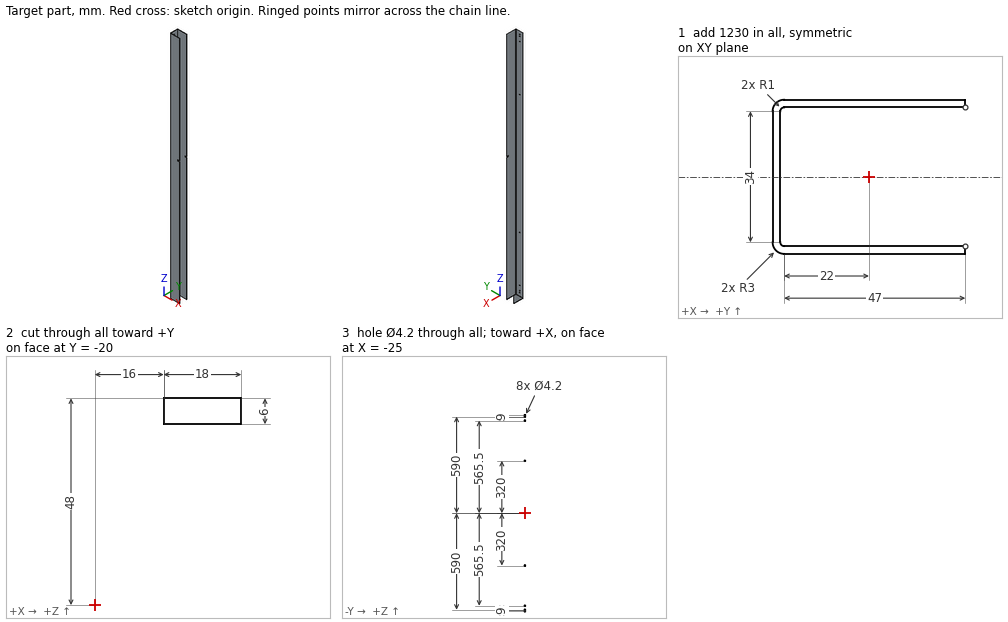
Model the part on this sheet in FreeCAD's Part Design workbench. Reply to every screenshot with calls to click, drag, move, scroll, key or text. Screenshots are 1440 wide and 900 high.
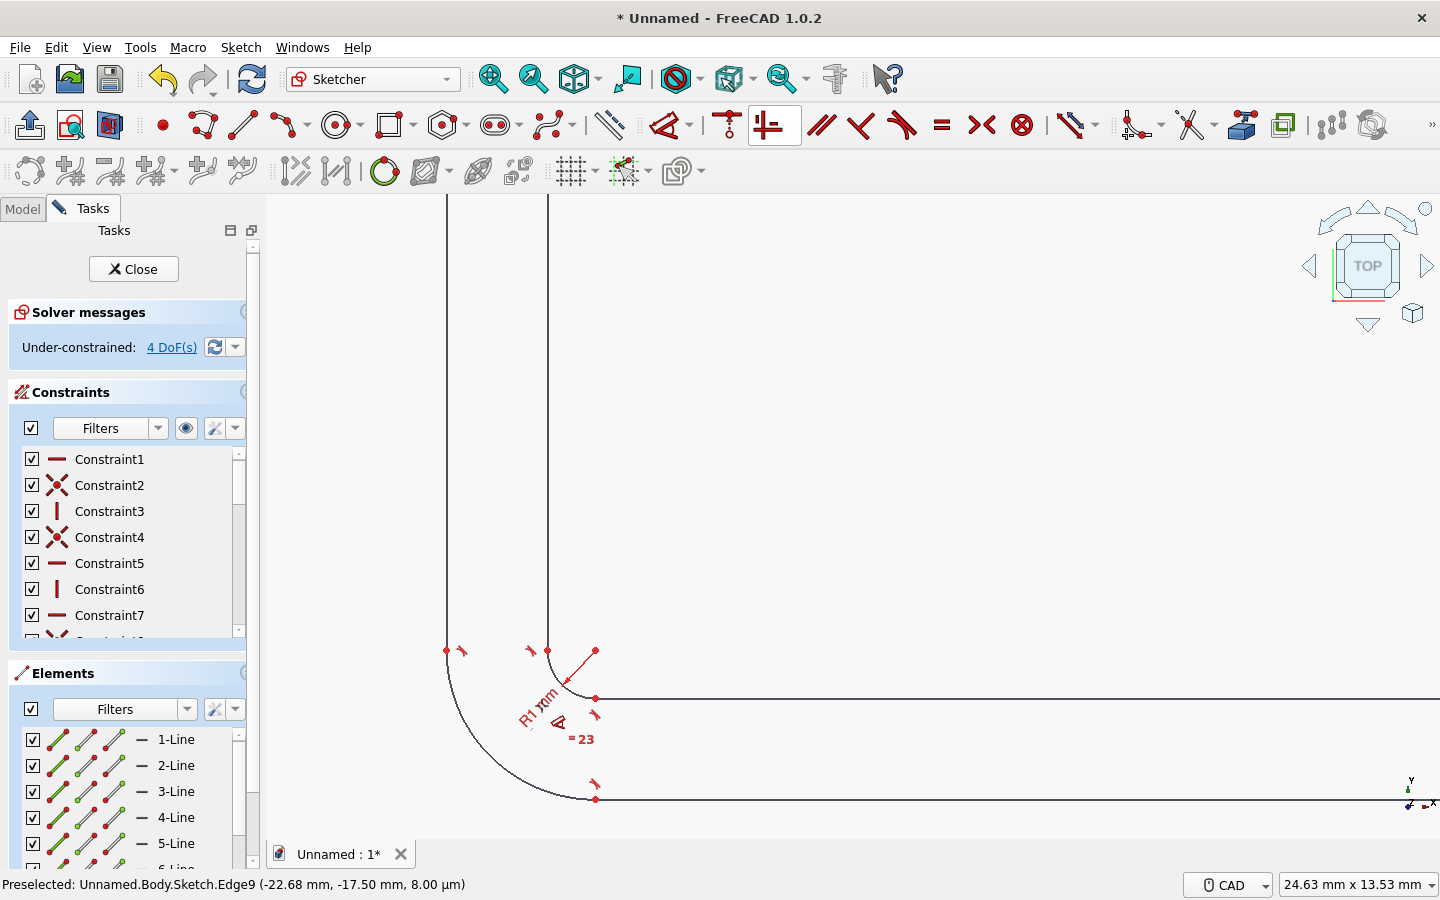
scroll(567, 686, down, 8)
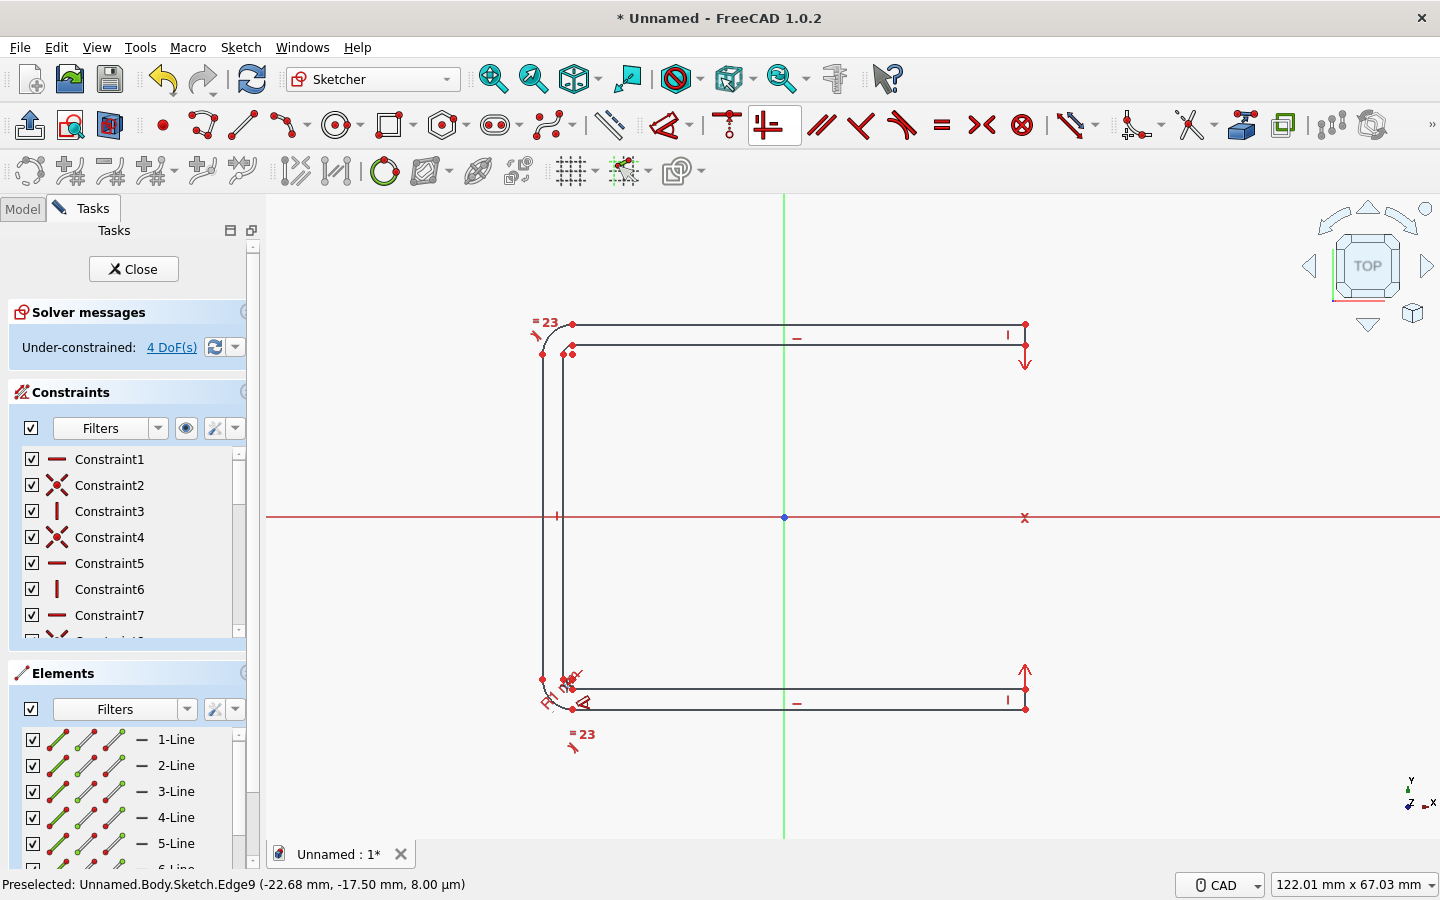
scroll(559, 328, up, 2)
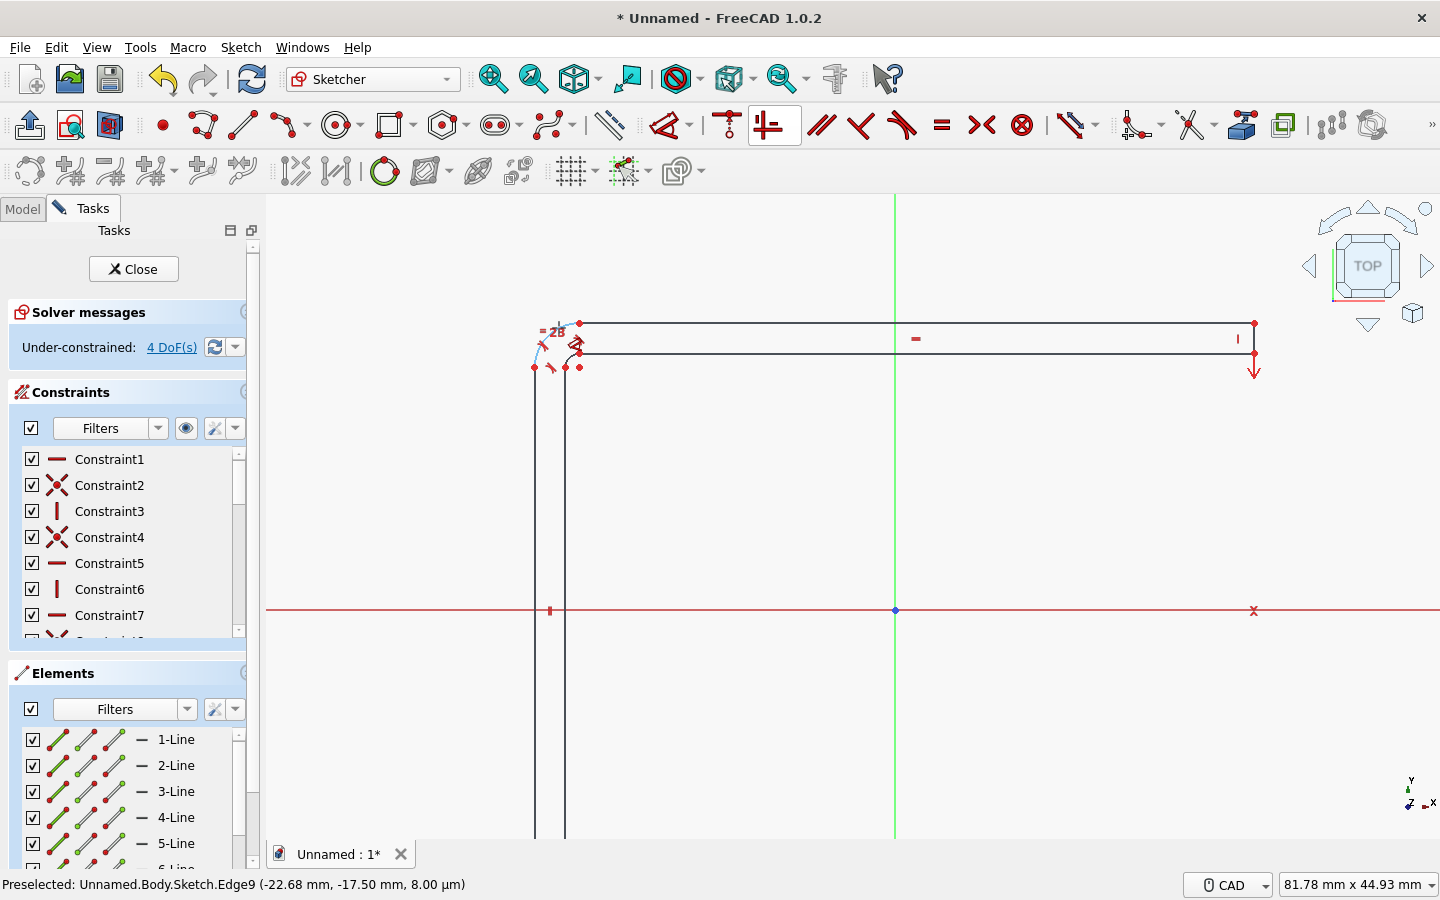
click(559, 328)
click(544, 300)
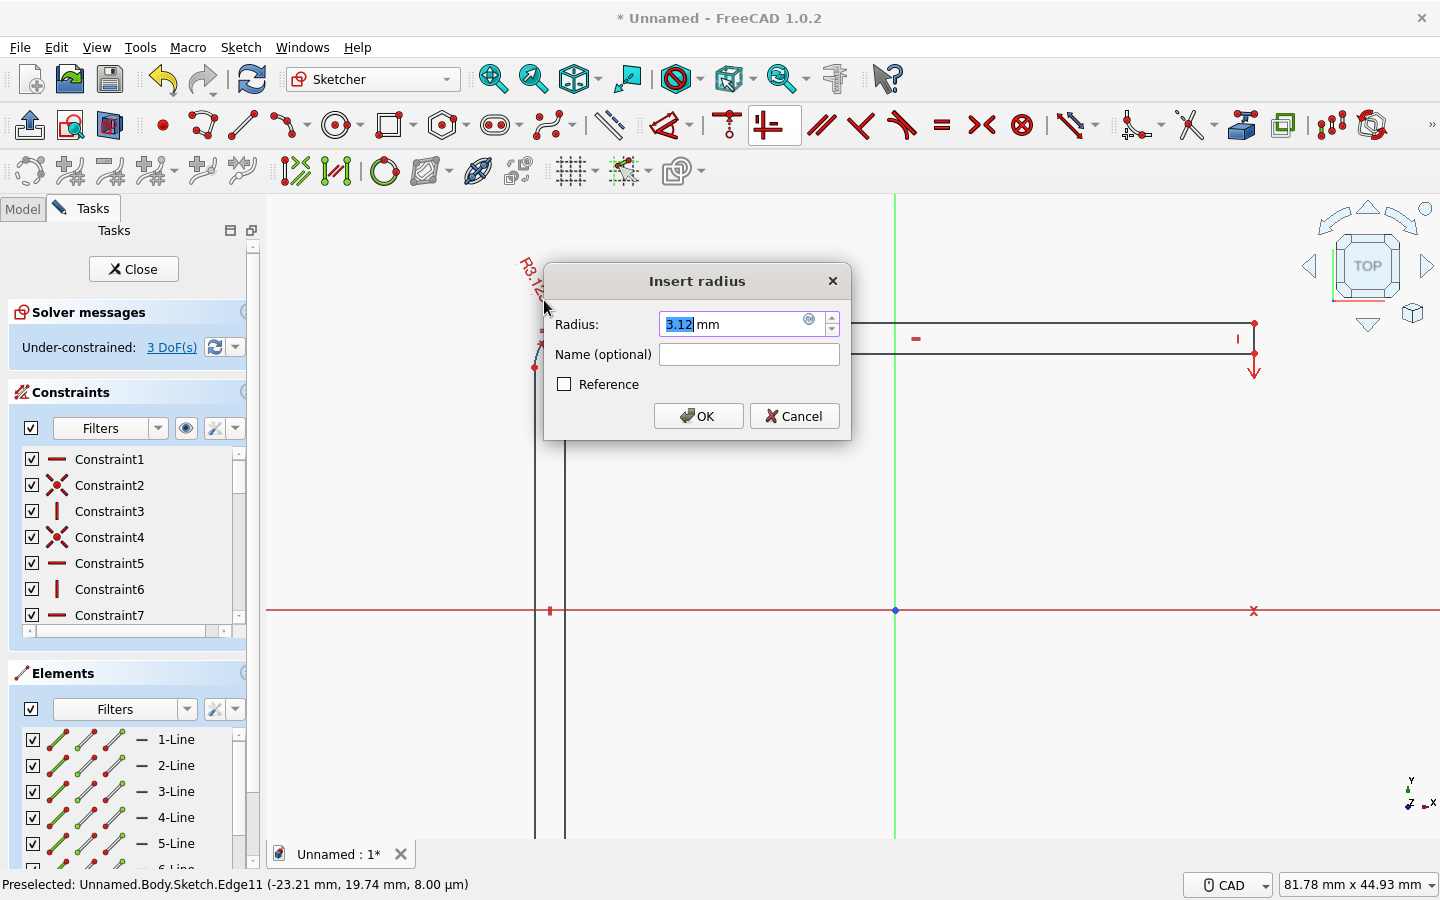
text(3)
key(Return)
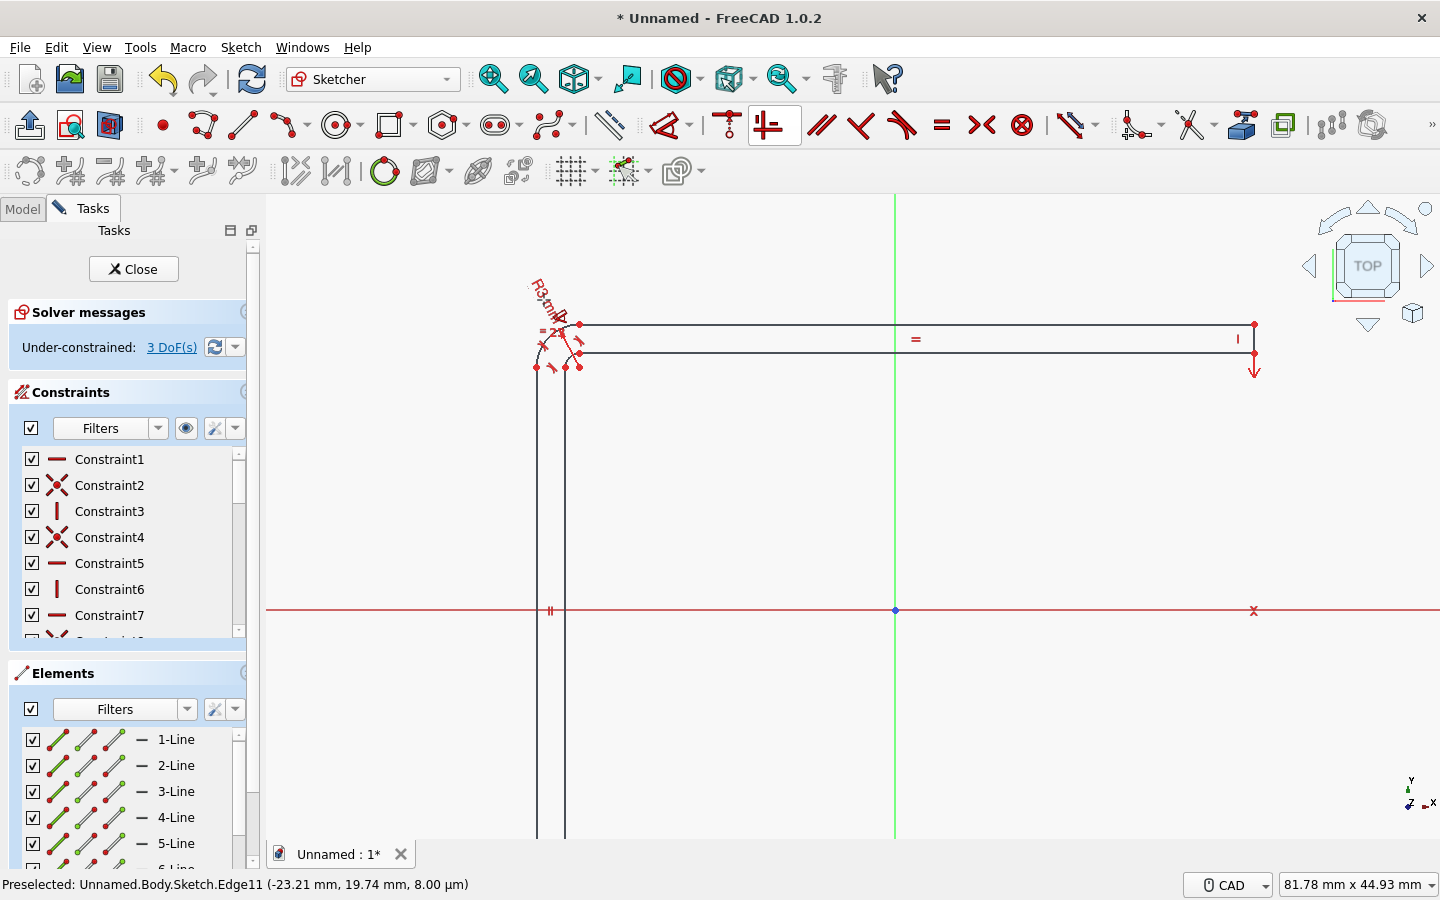
scroll(560, 326, down, 2)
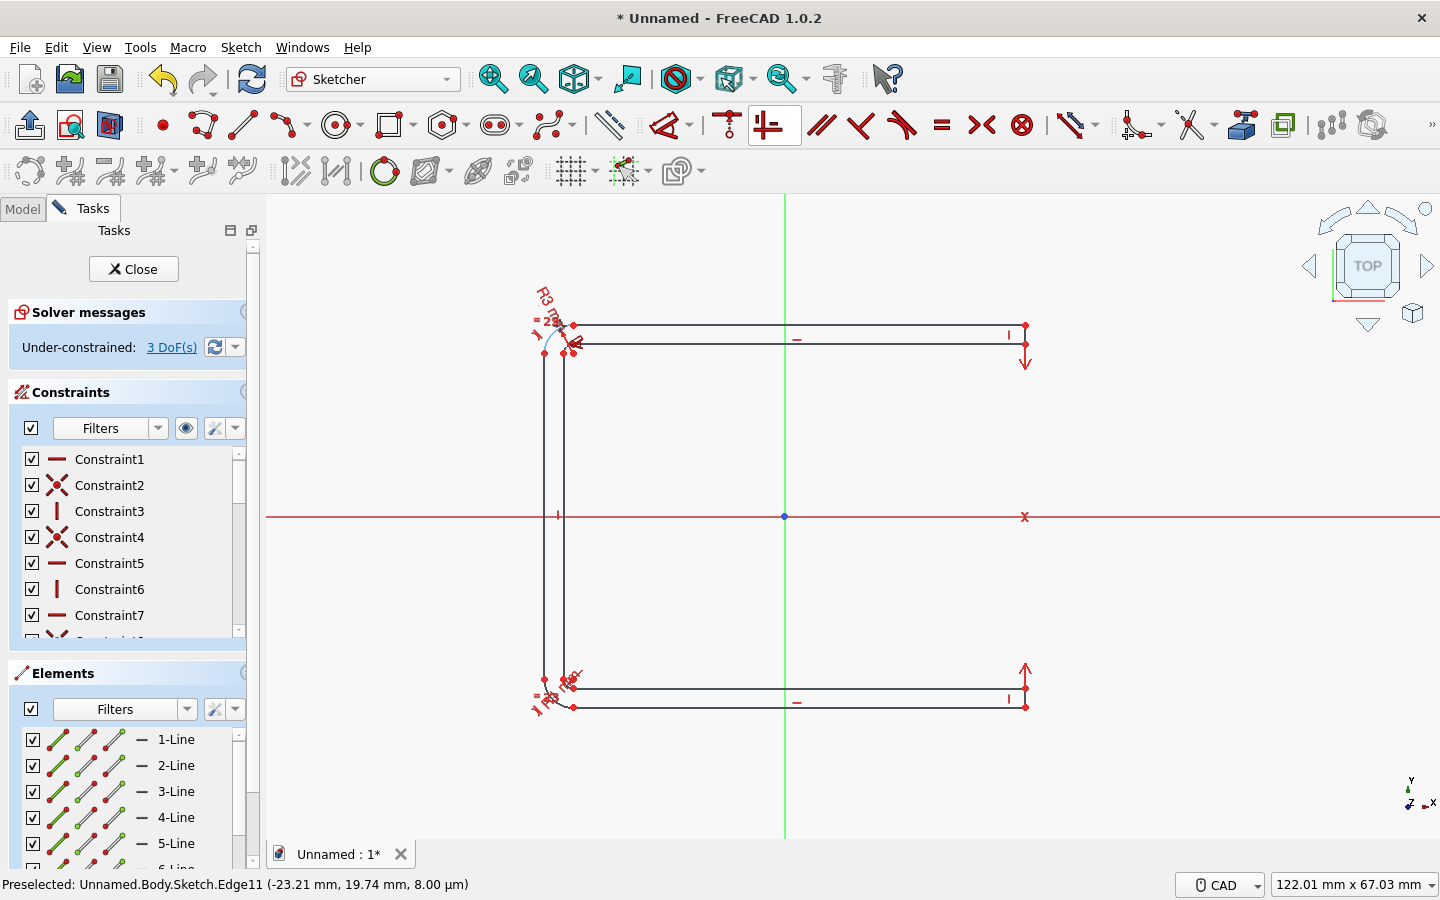
click(709, 708)
click(799, 742)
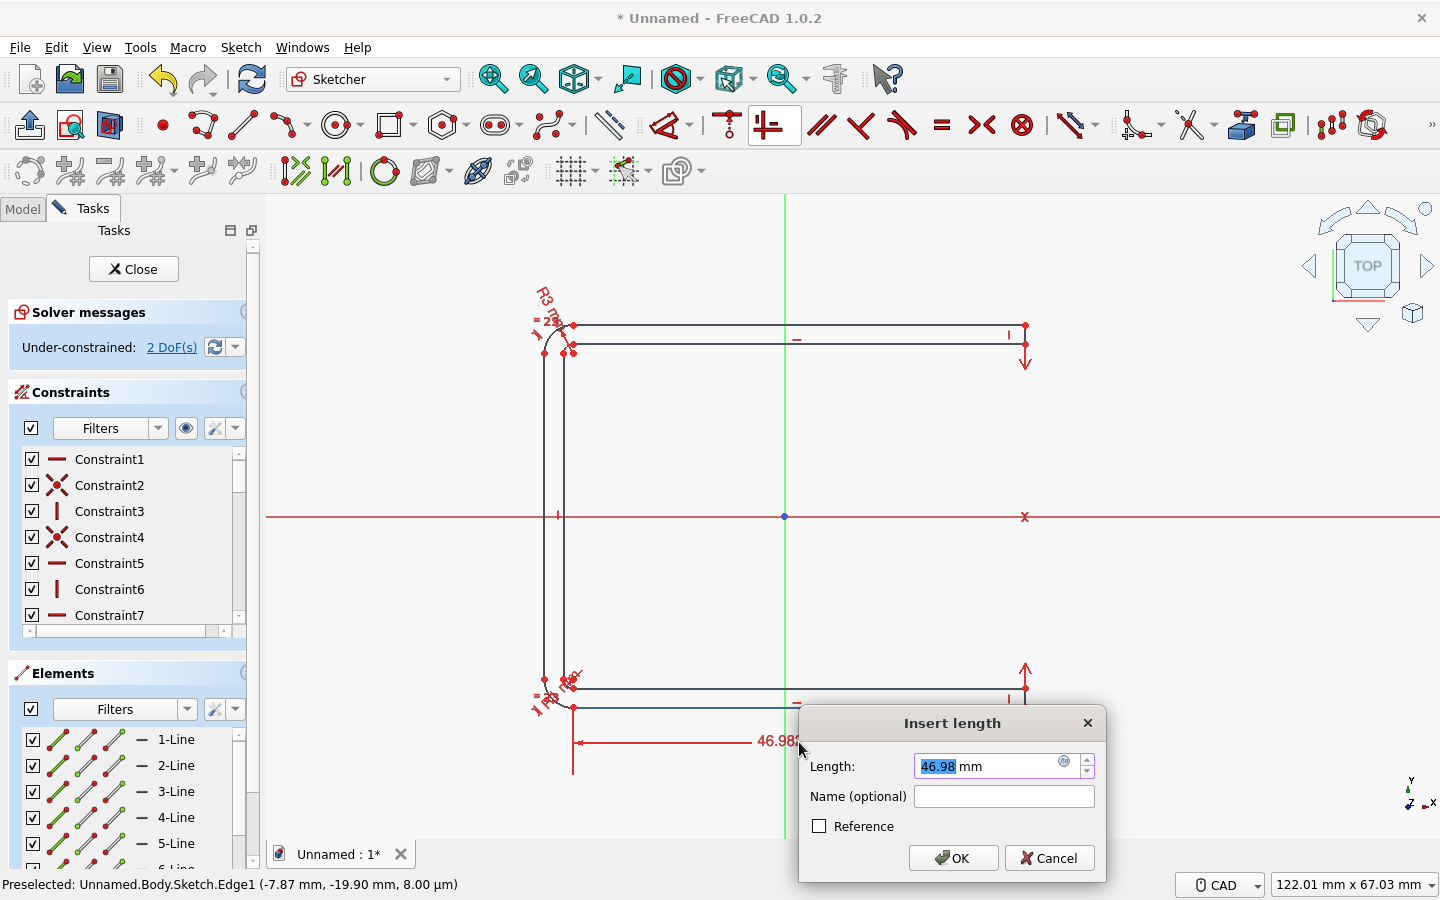
text(47)
key(Return)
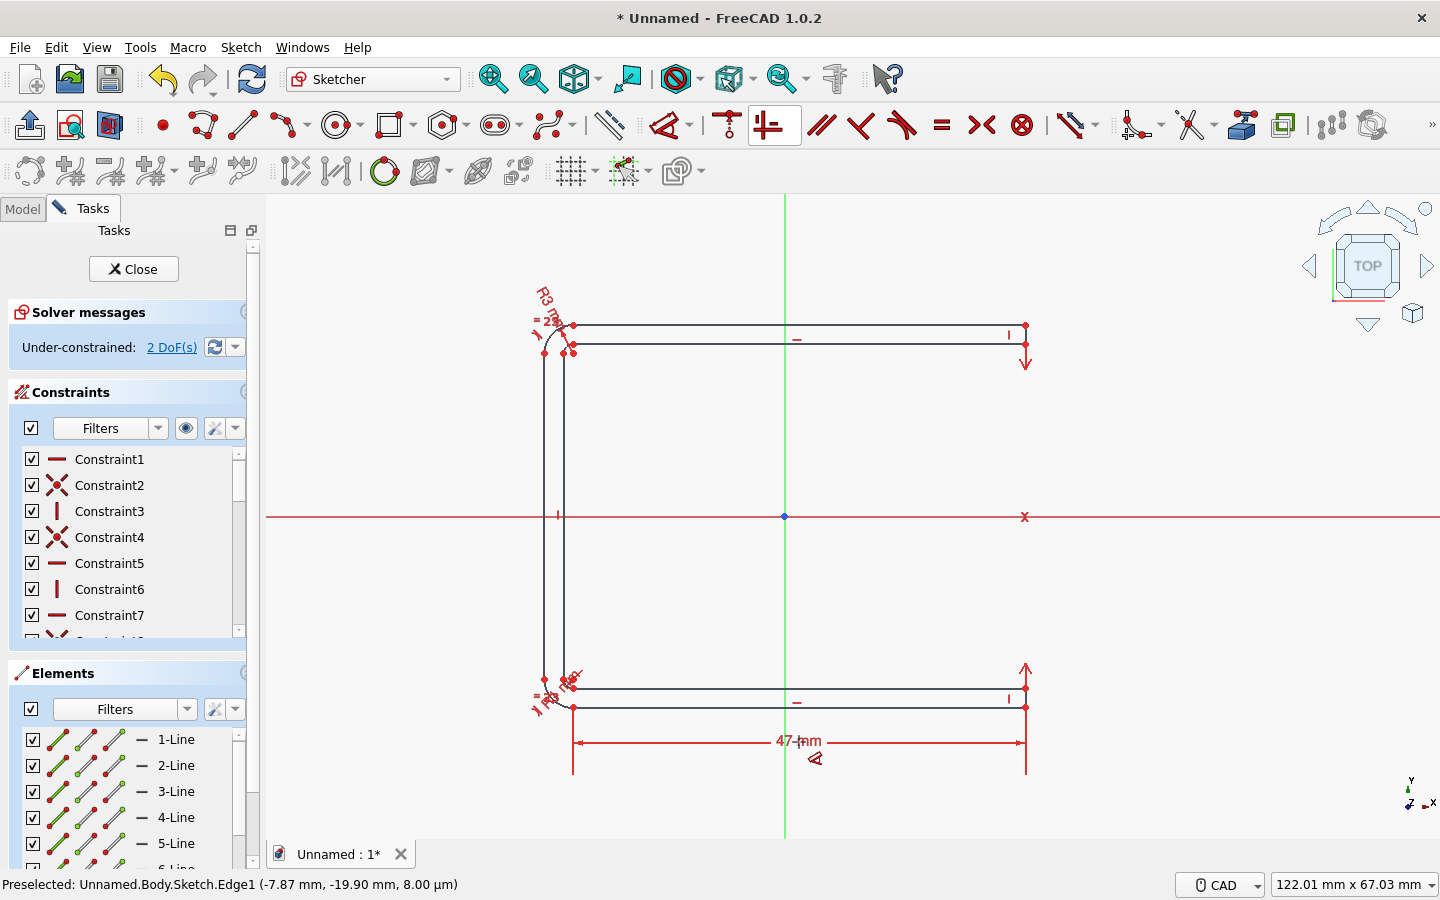
click(564, 582)
click(530, 442)